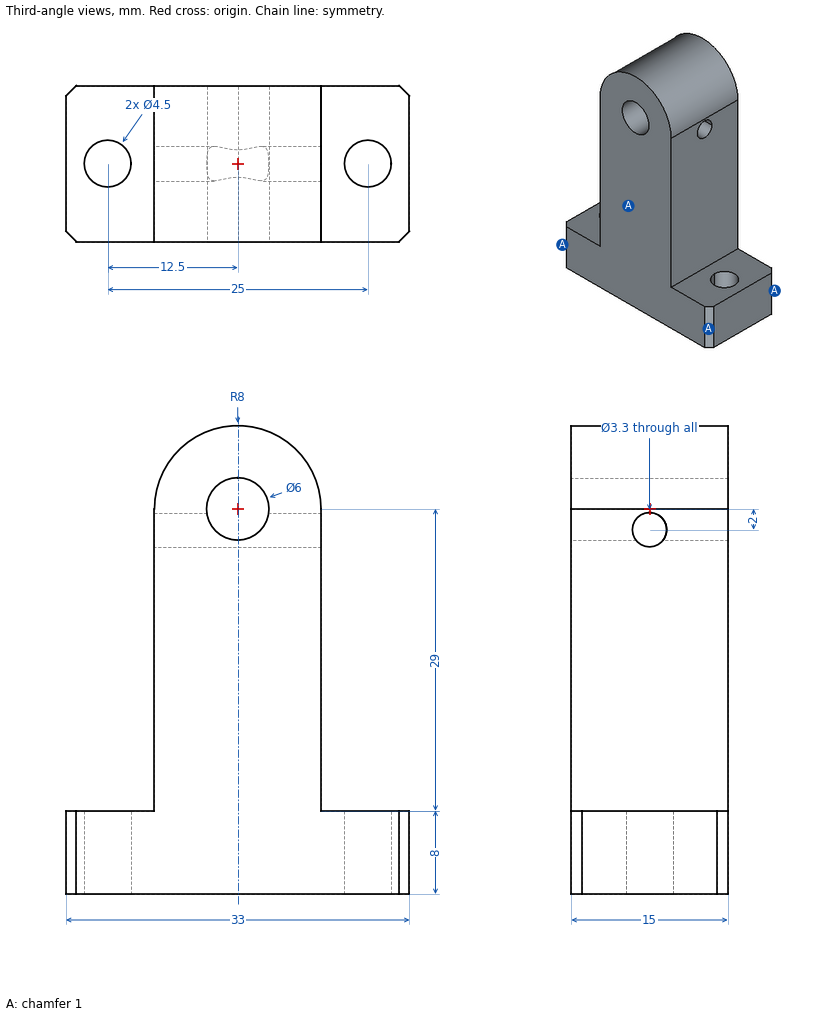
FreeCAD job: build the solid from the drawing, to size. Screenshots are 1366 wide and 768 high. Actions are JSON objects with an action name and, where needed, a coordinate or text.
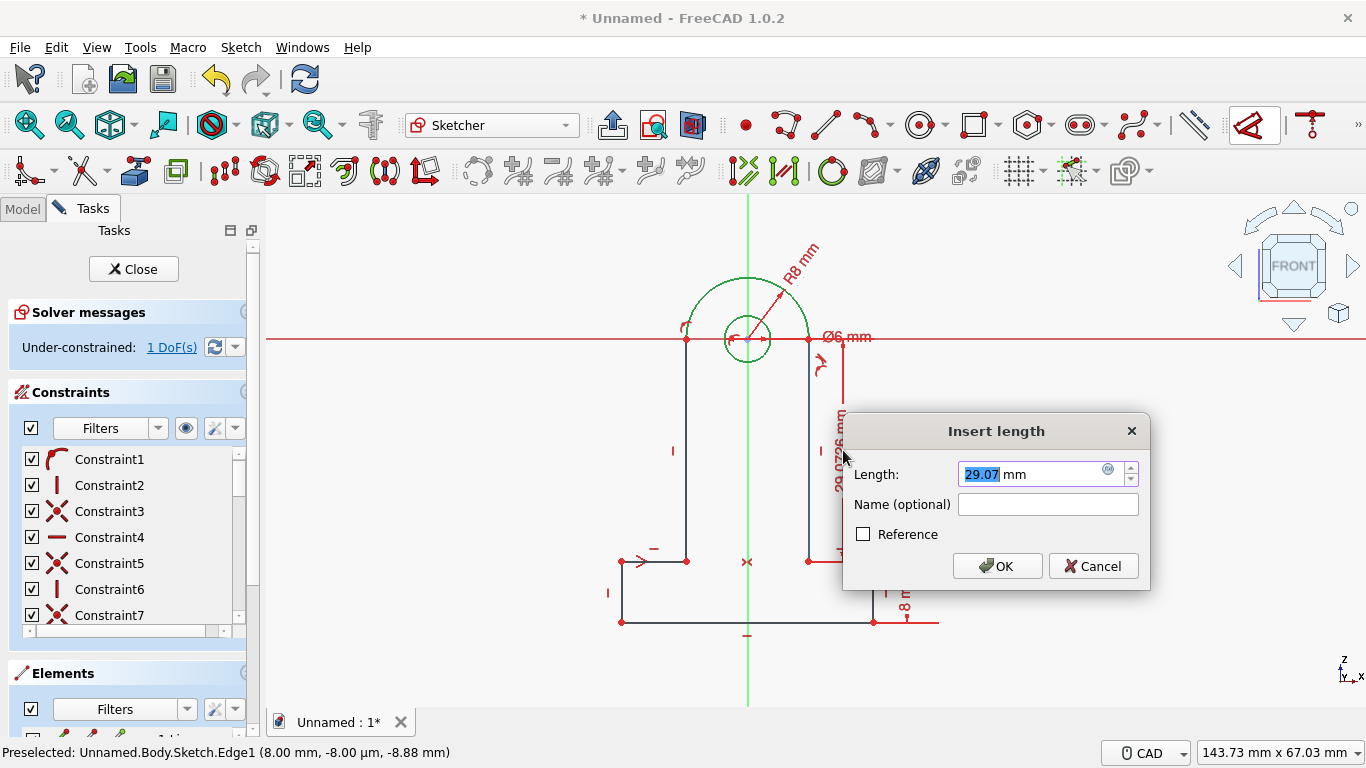
{"action": "type", "text": "29"}
{"action": "key", "text": "Return"}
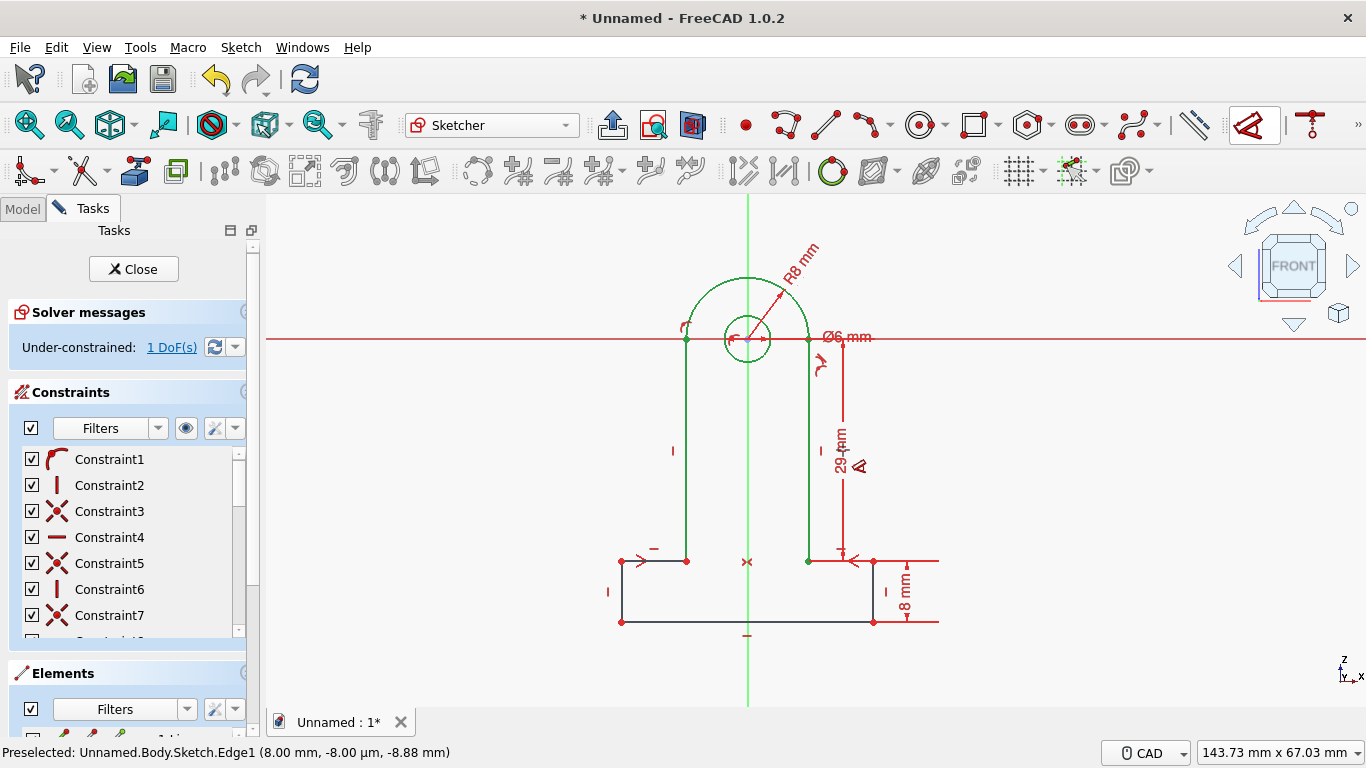
{"action": "left_click", "coordinate": [798, 622]}
{"action": "left_click", "coordinate": [690, 656]}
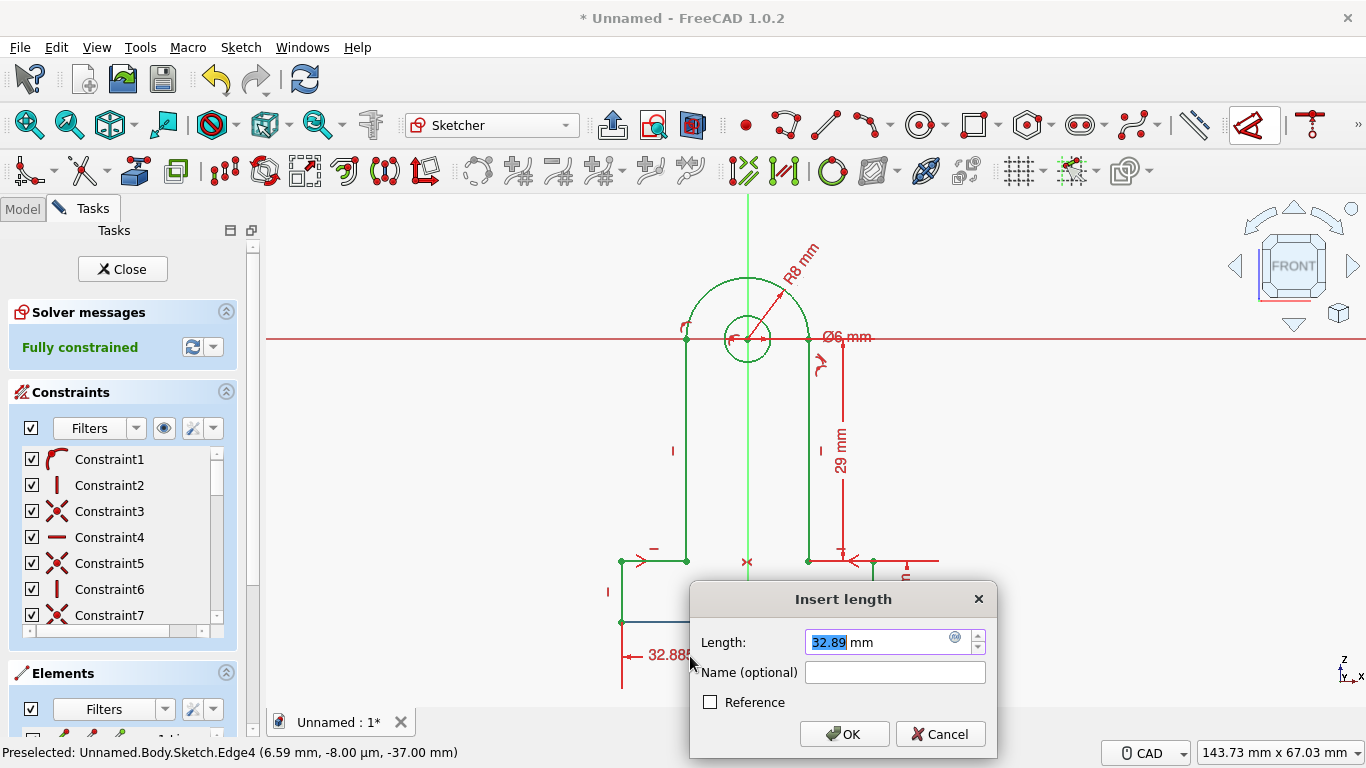
{"action": "type", "text": "33"}
{"action": "key", "text": "Return"}
{"action": "key", "text": "Escape"}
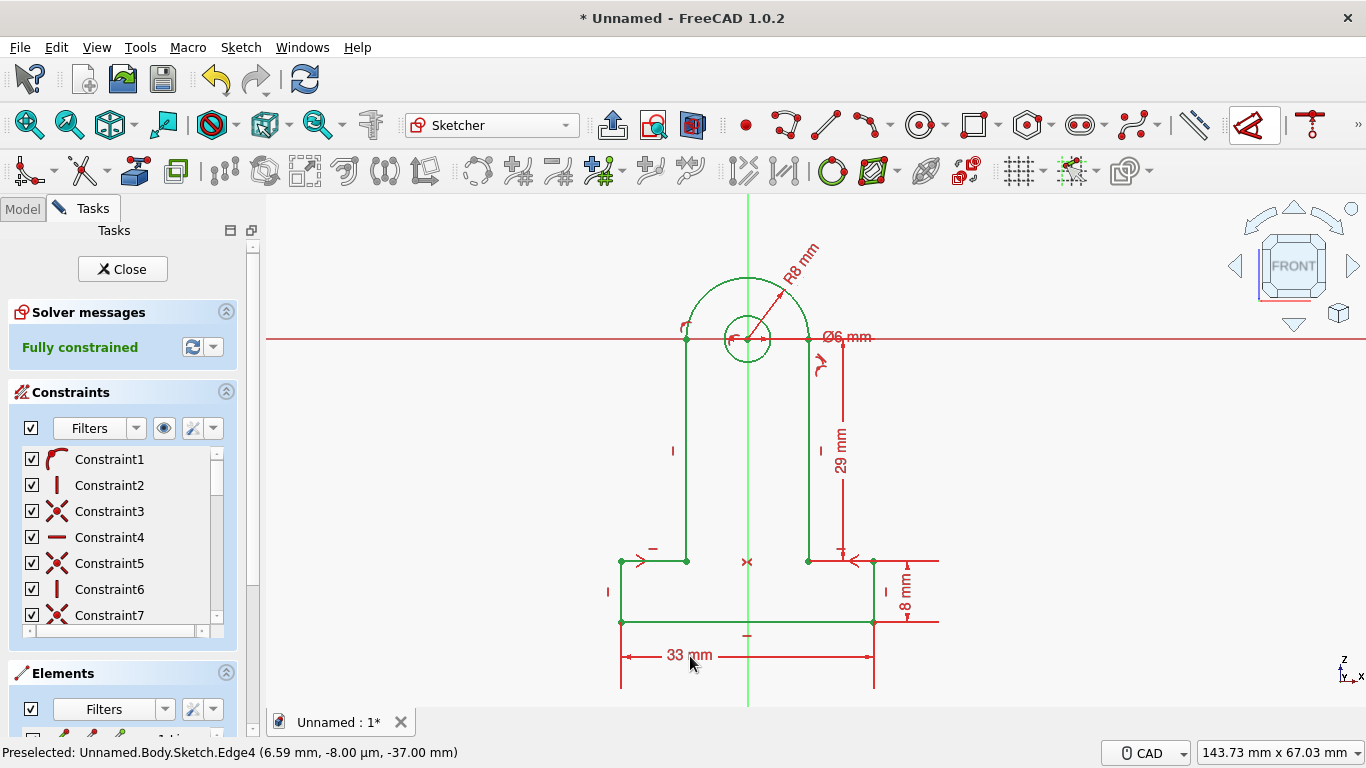
{"action": "left_click", "coordinate": [123, 269]}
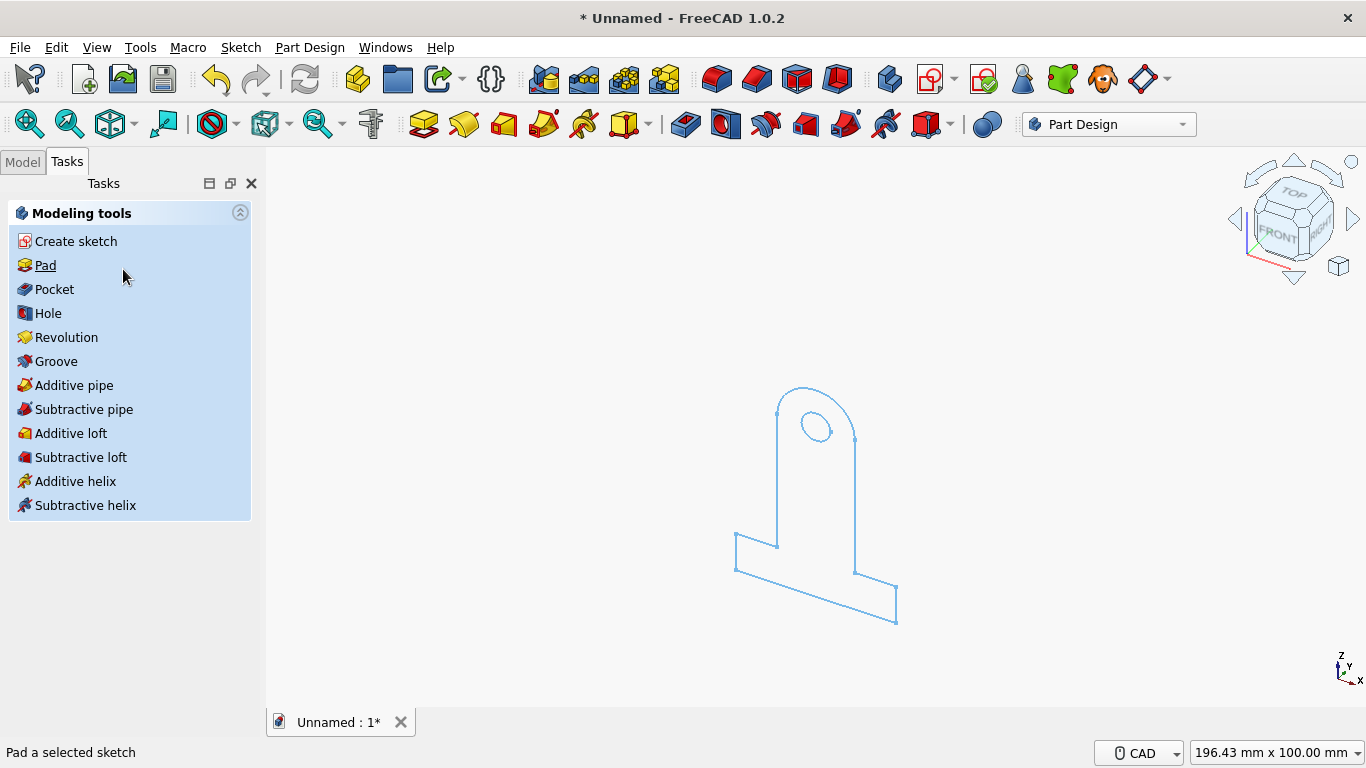
{"action": "left_click", "coordinate": [424, 124]}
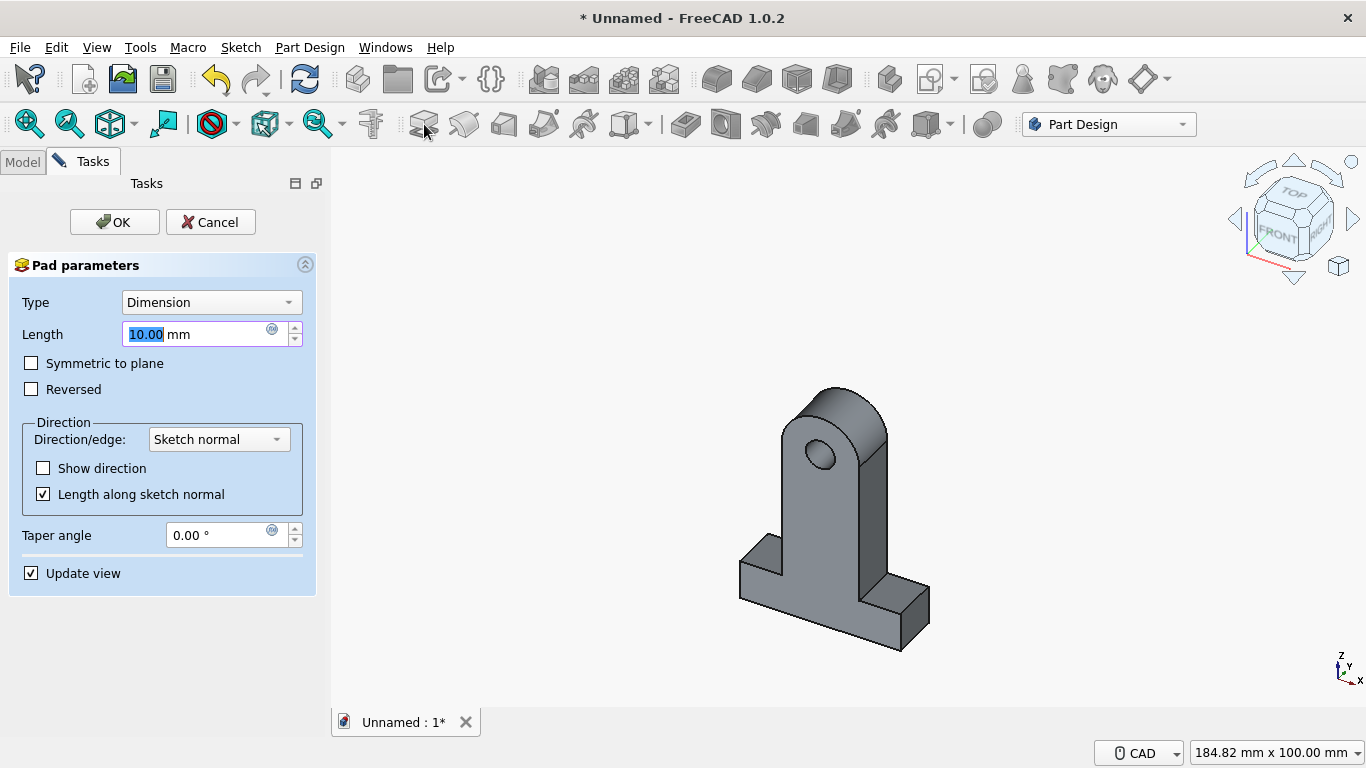
{"action": "type", "text": "15"}
{"action": "key", "text": "Tab"}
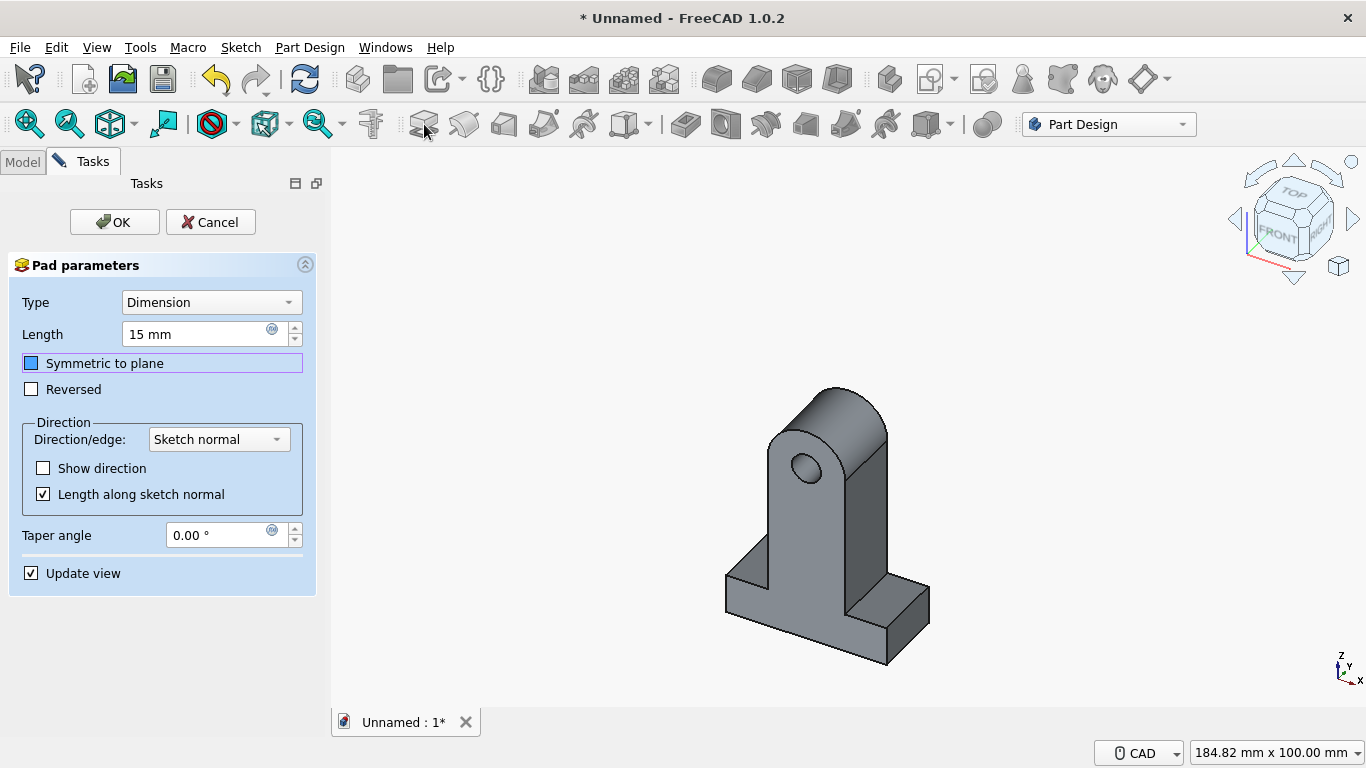
{"action": "left_click", "coordinate": [30, 363]}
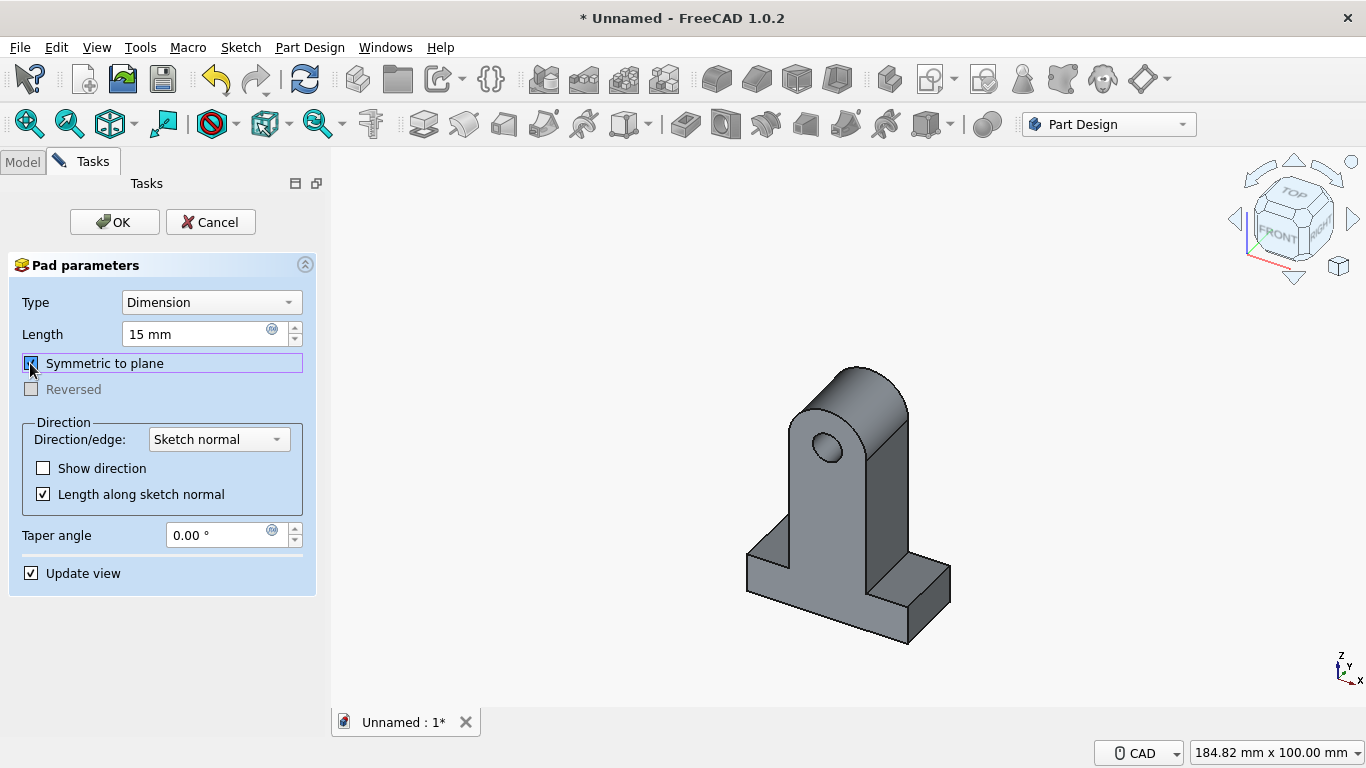
{"action": "left_click", "coordinate": [115, 222]}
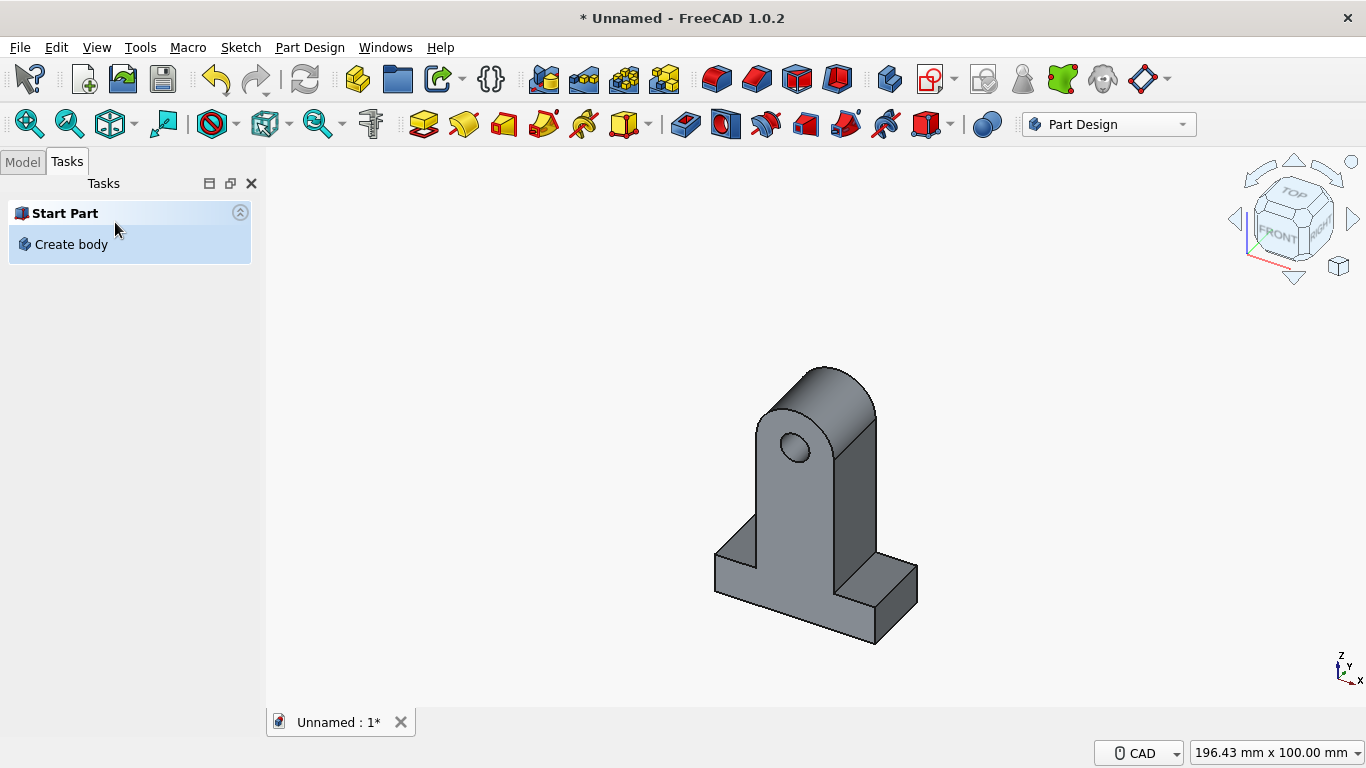
{"action": "left_click", "coordinate": [855, 486]}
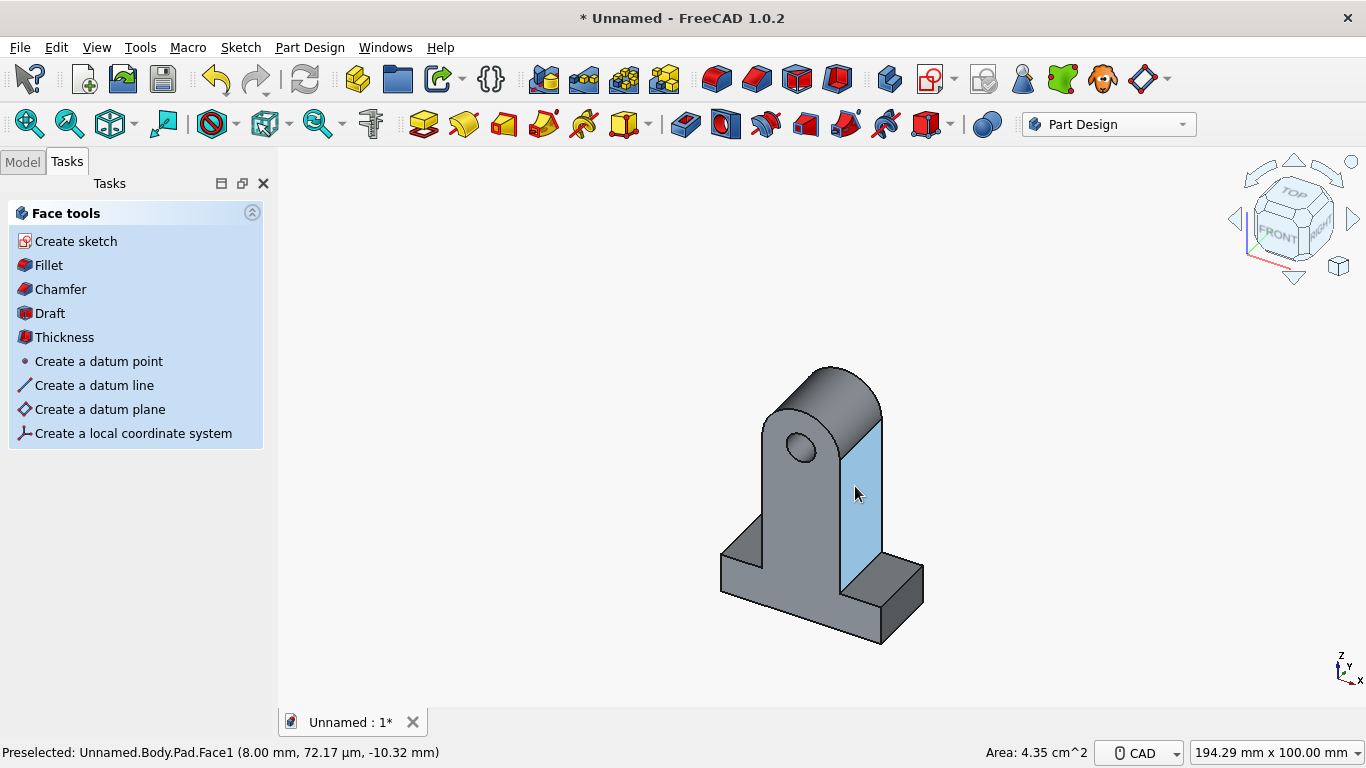
{"action": "left_click", "coordinate": [930, 80]}